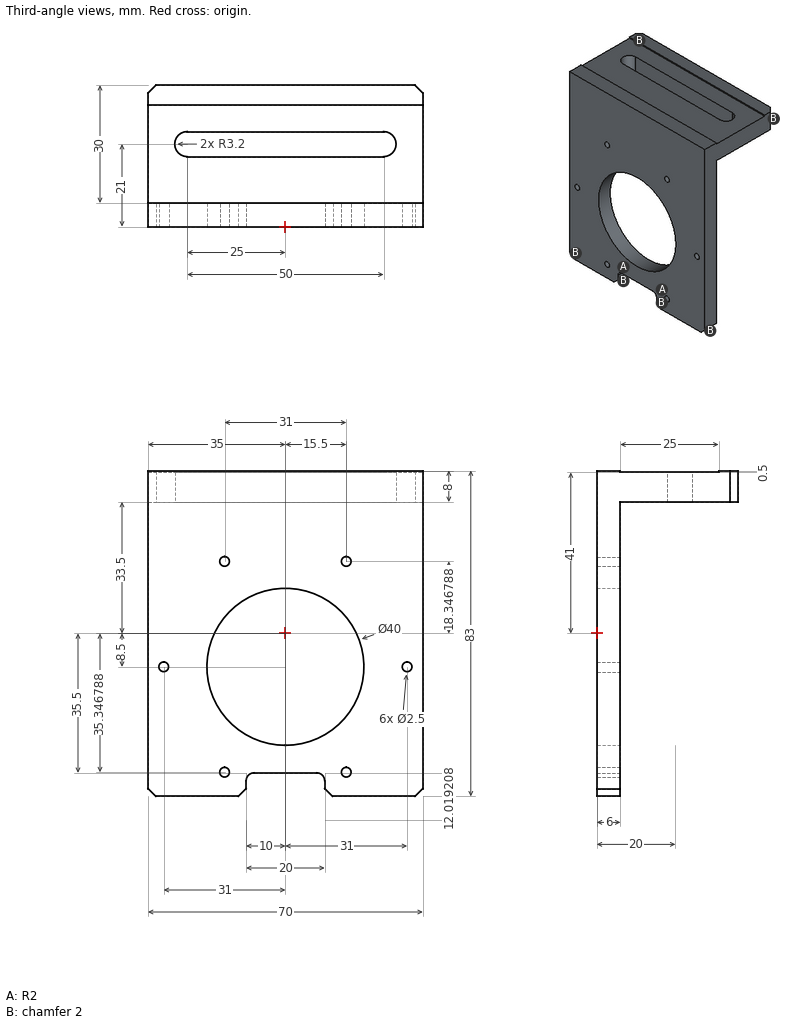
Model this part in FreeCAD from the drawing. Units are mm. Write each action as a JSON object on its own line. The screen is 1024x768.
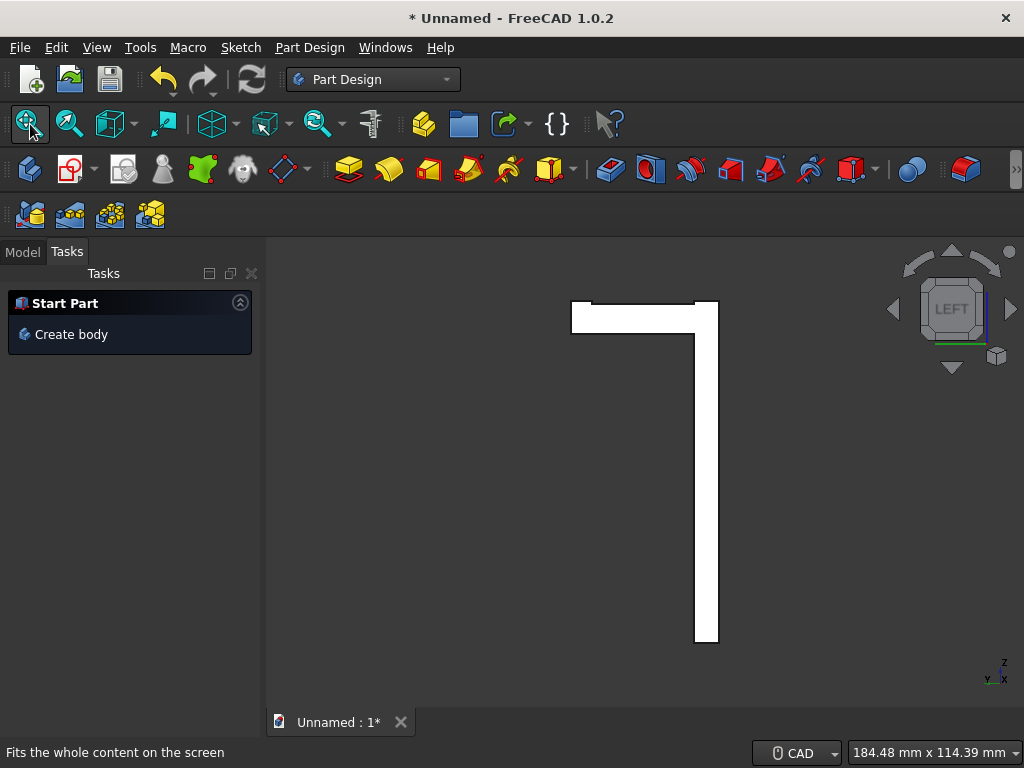
{"action": "key", "text": "0"}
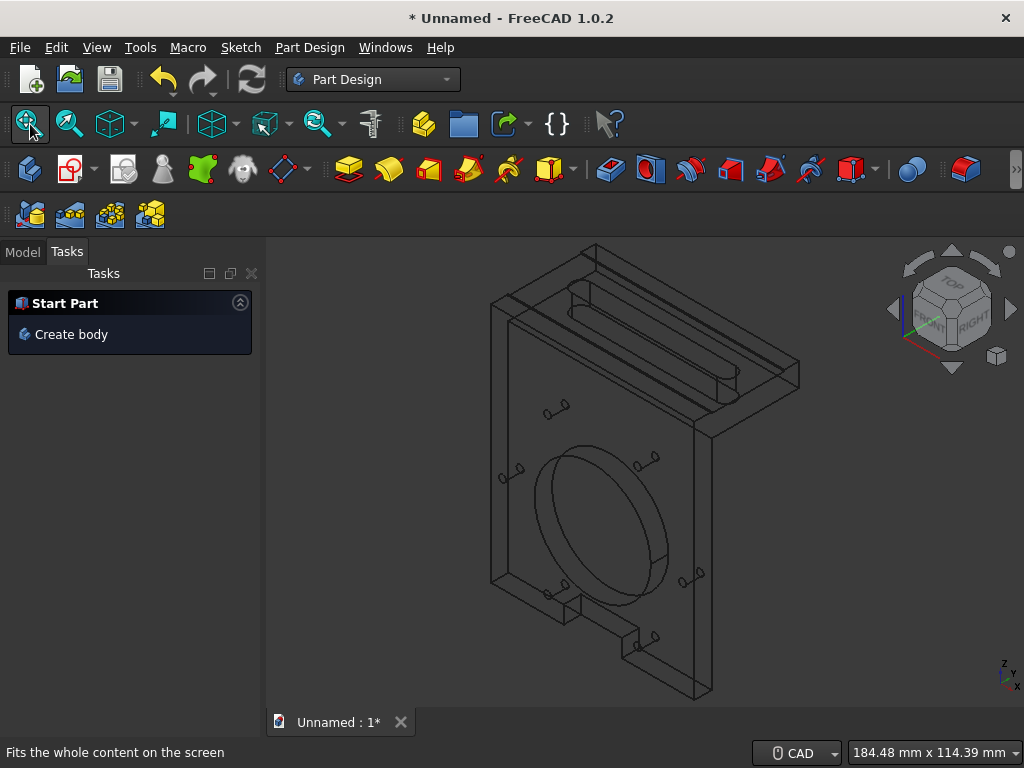
{"action": "left_click", "coordinate": [572, 598]}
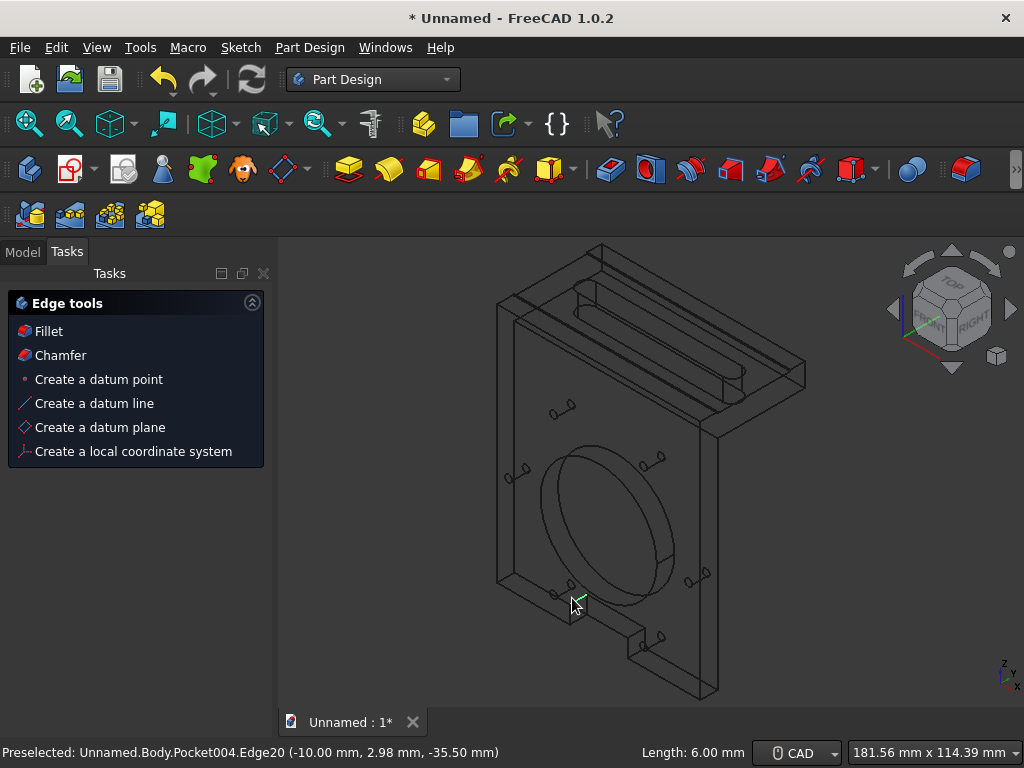
{"action": "left_click", "coordinate": [636, 632], "text": "ctrl"}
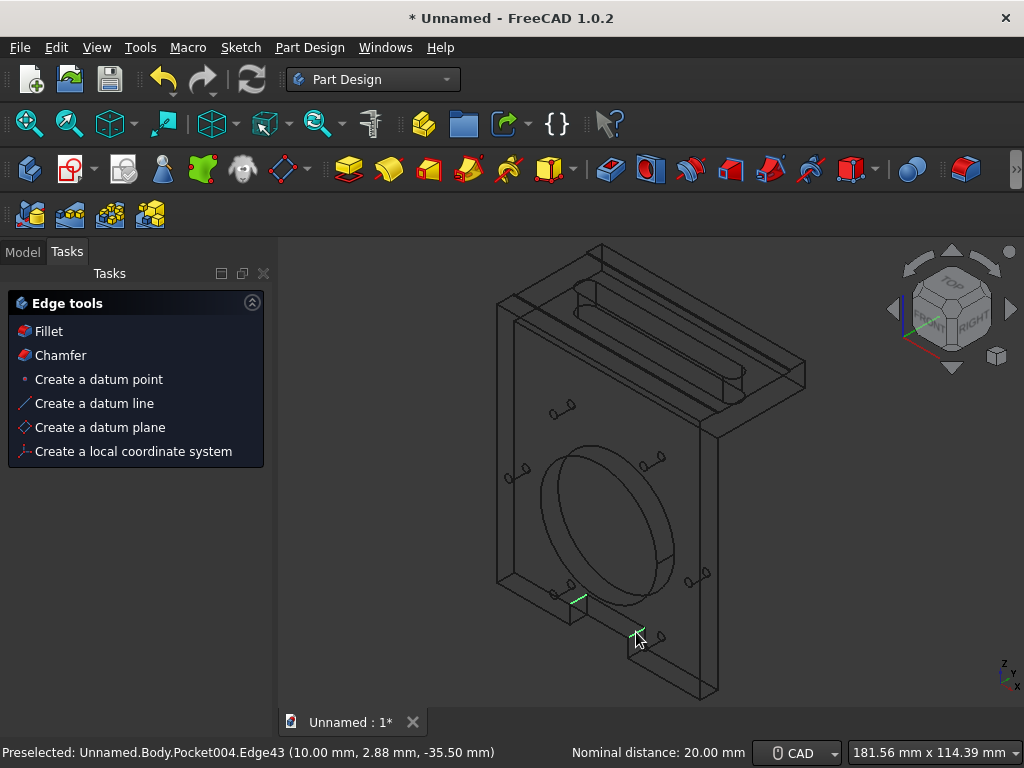
{"action": "key", "text": "v 1"}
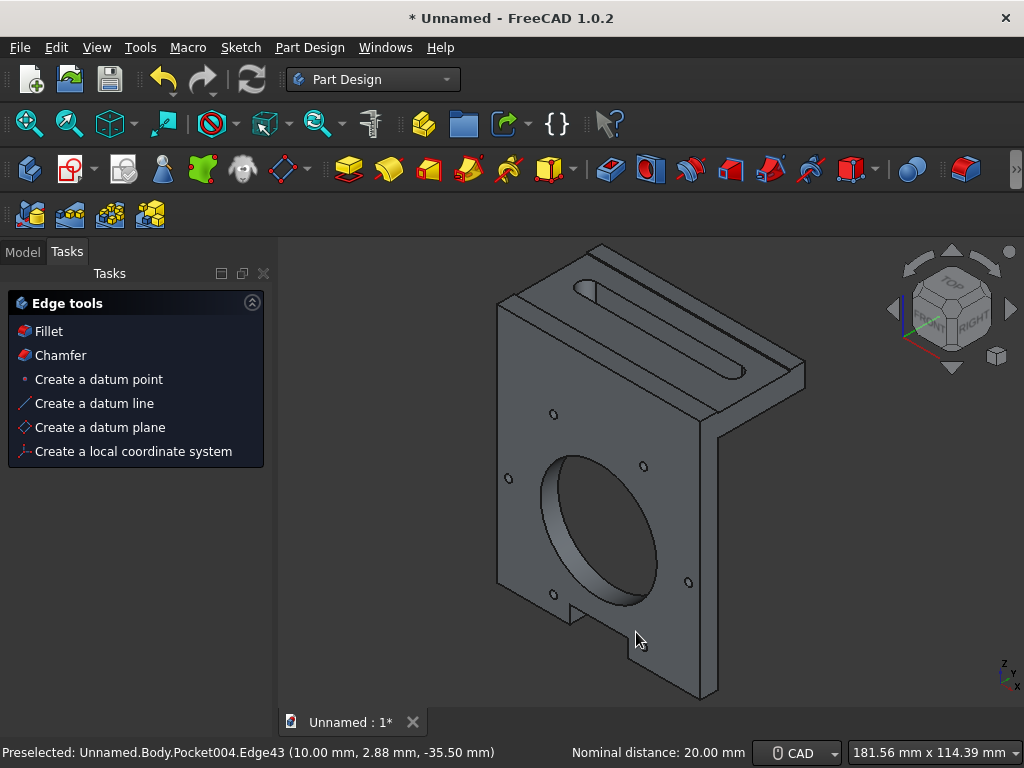
{"action": "left_click", "coordinate": [966, 170]}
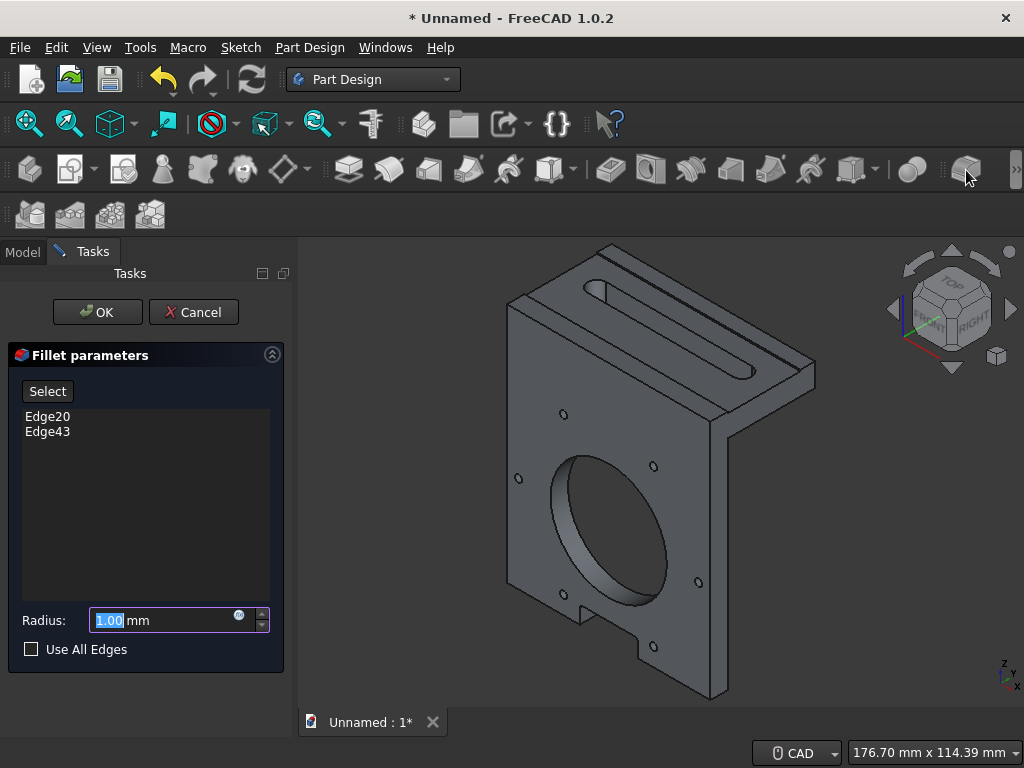
{"action": "type", "text": "2"}
{"action": "key", "text": "Tab"}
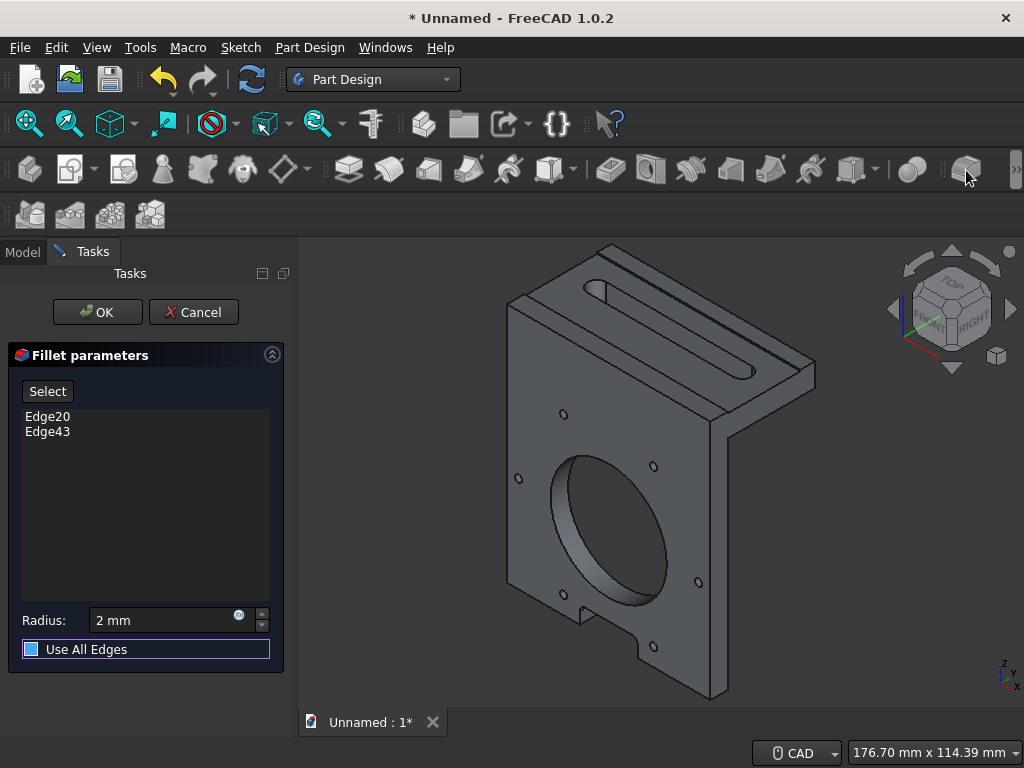
{"action": "left_click", "coordinate": [98, 312]}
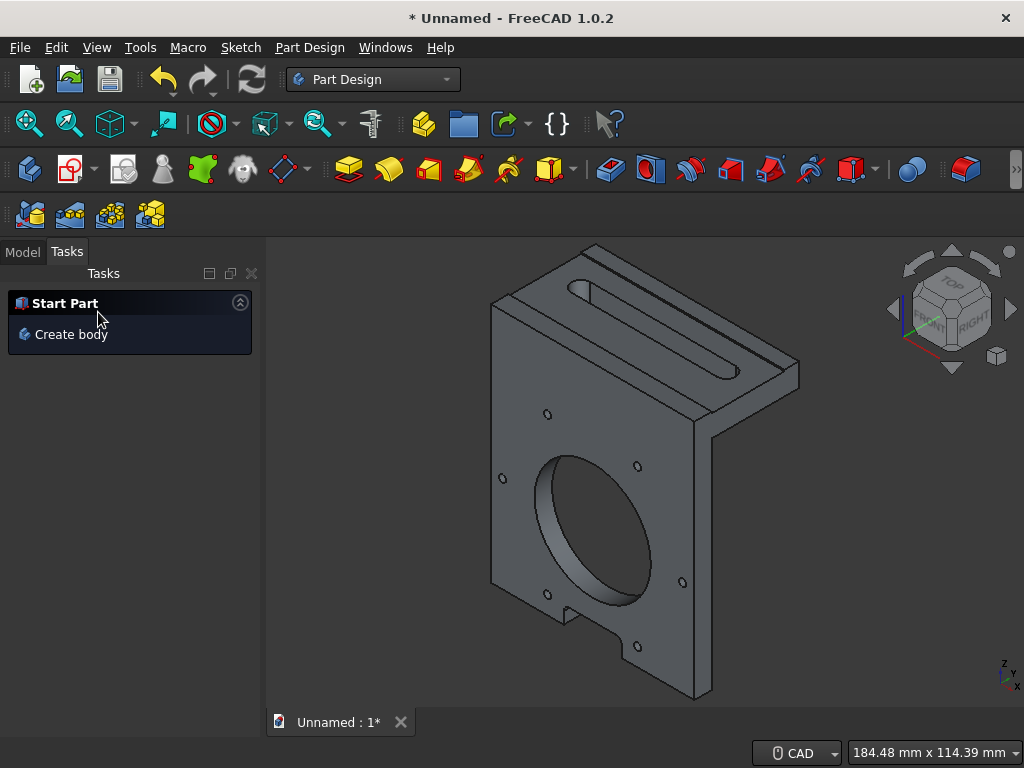
{"action": "key", "text": "2"}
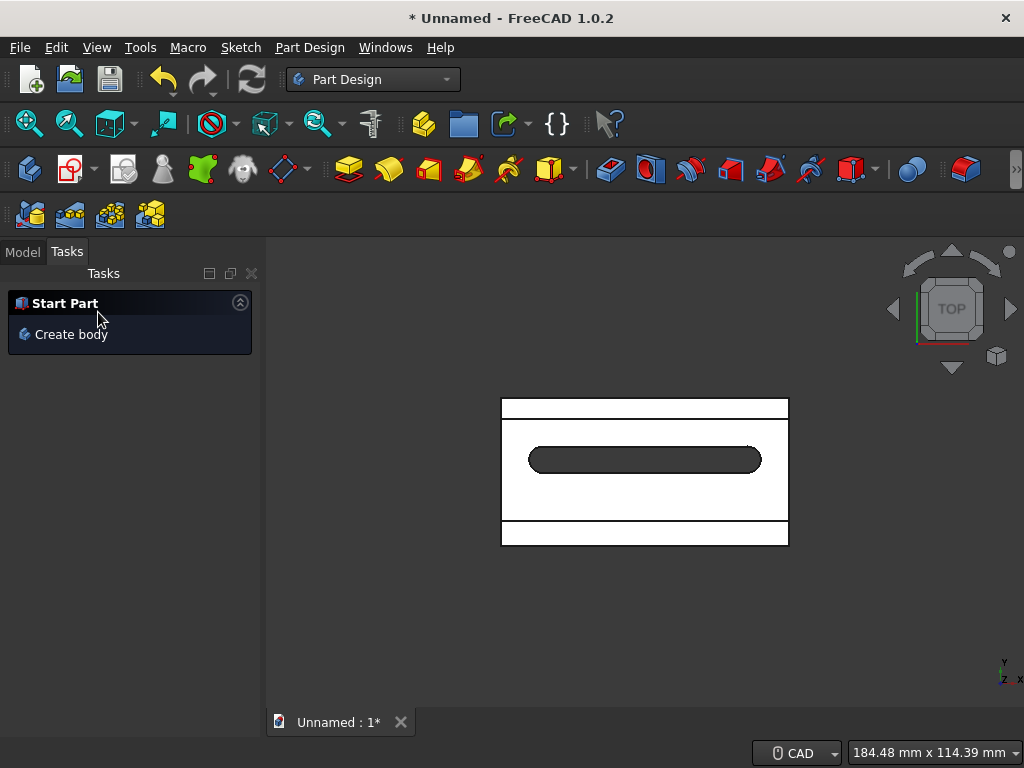
{"action": "left_click", "coordinate": [30, 124]}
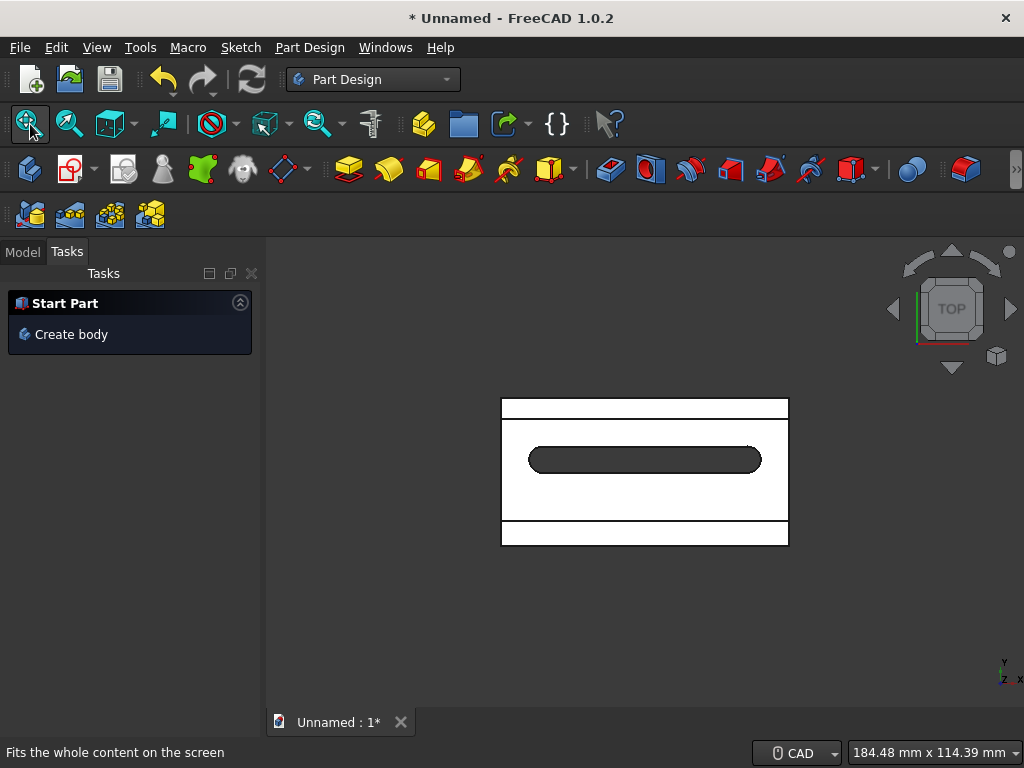
{"action": "key", "text": "0"}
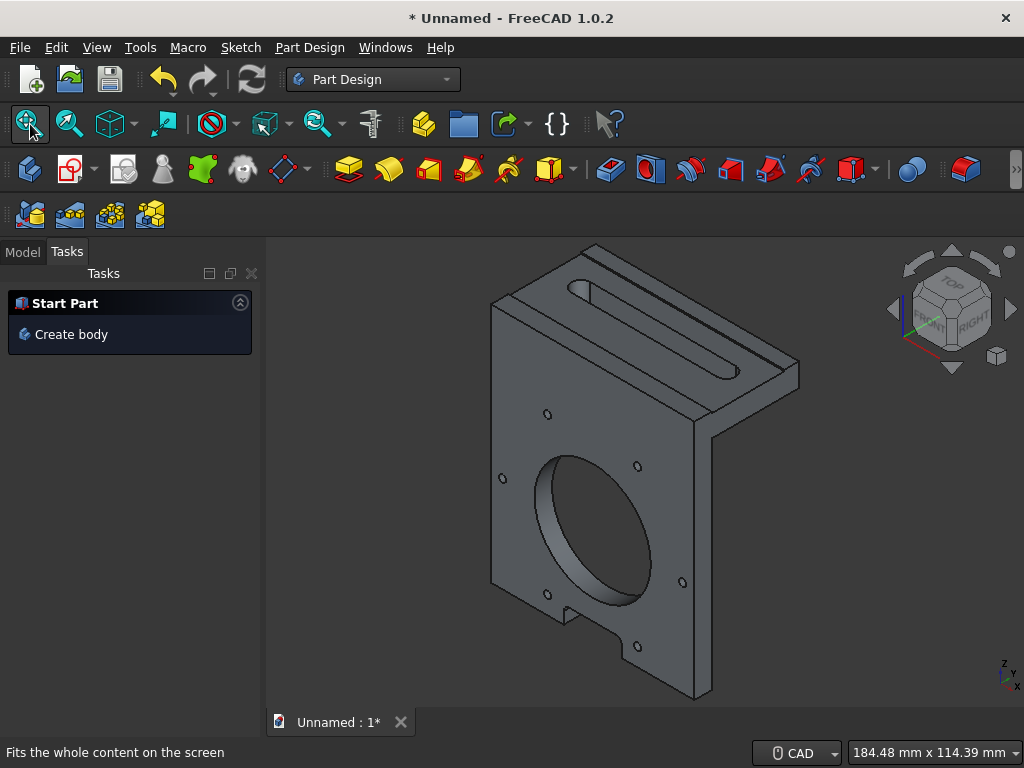
{"action": "key", "text": "1"}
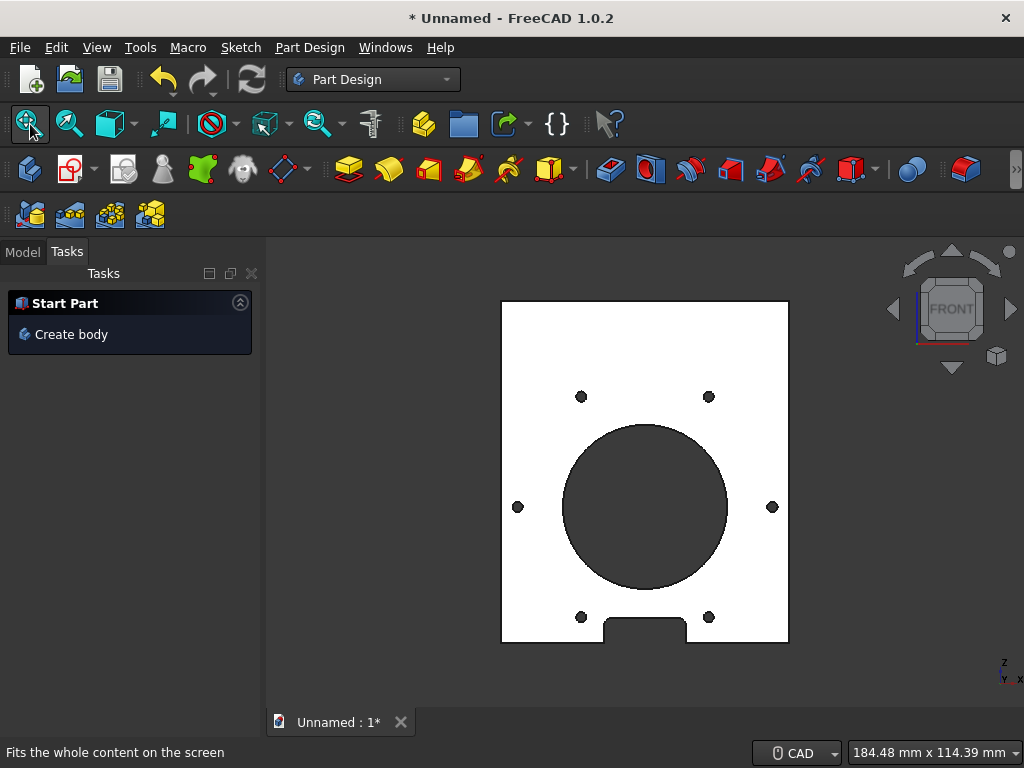
{"action": "key", "text": "3"}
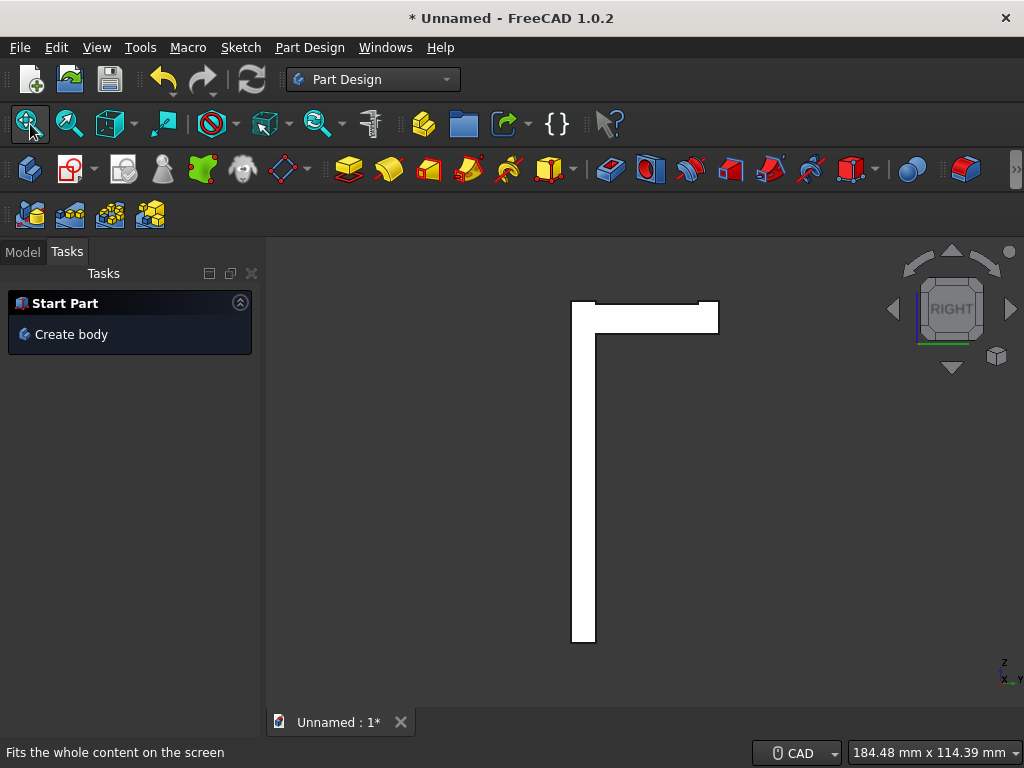
{"action": "left_click", "coordinate": [719, 317]}